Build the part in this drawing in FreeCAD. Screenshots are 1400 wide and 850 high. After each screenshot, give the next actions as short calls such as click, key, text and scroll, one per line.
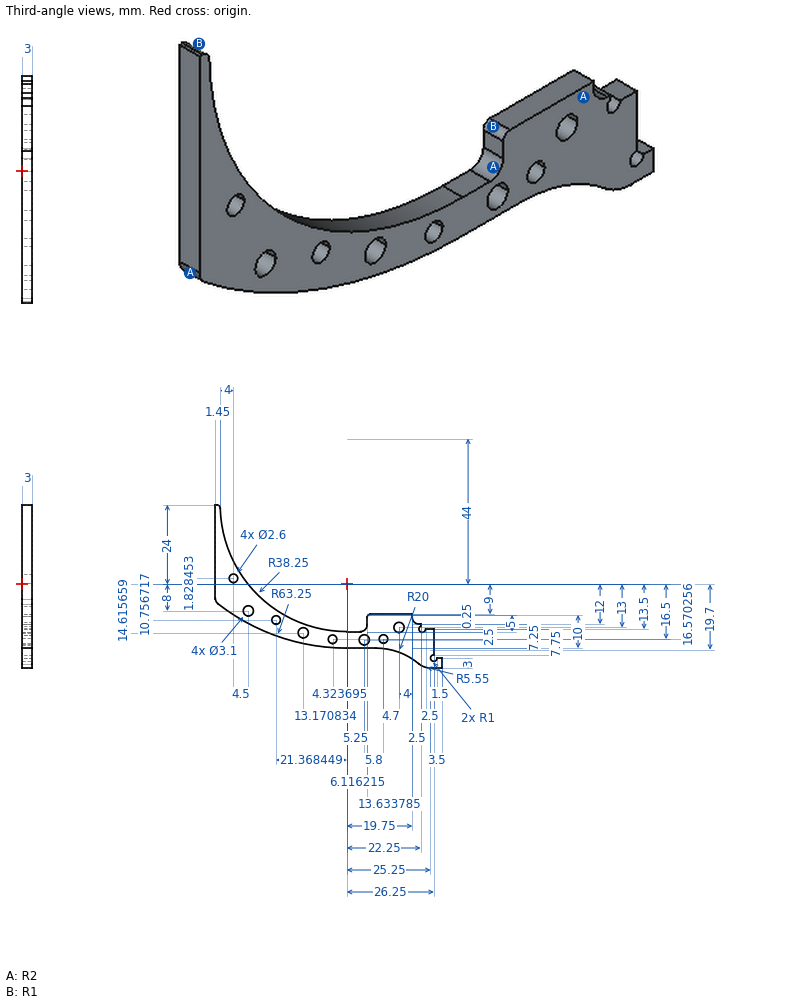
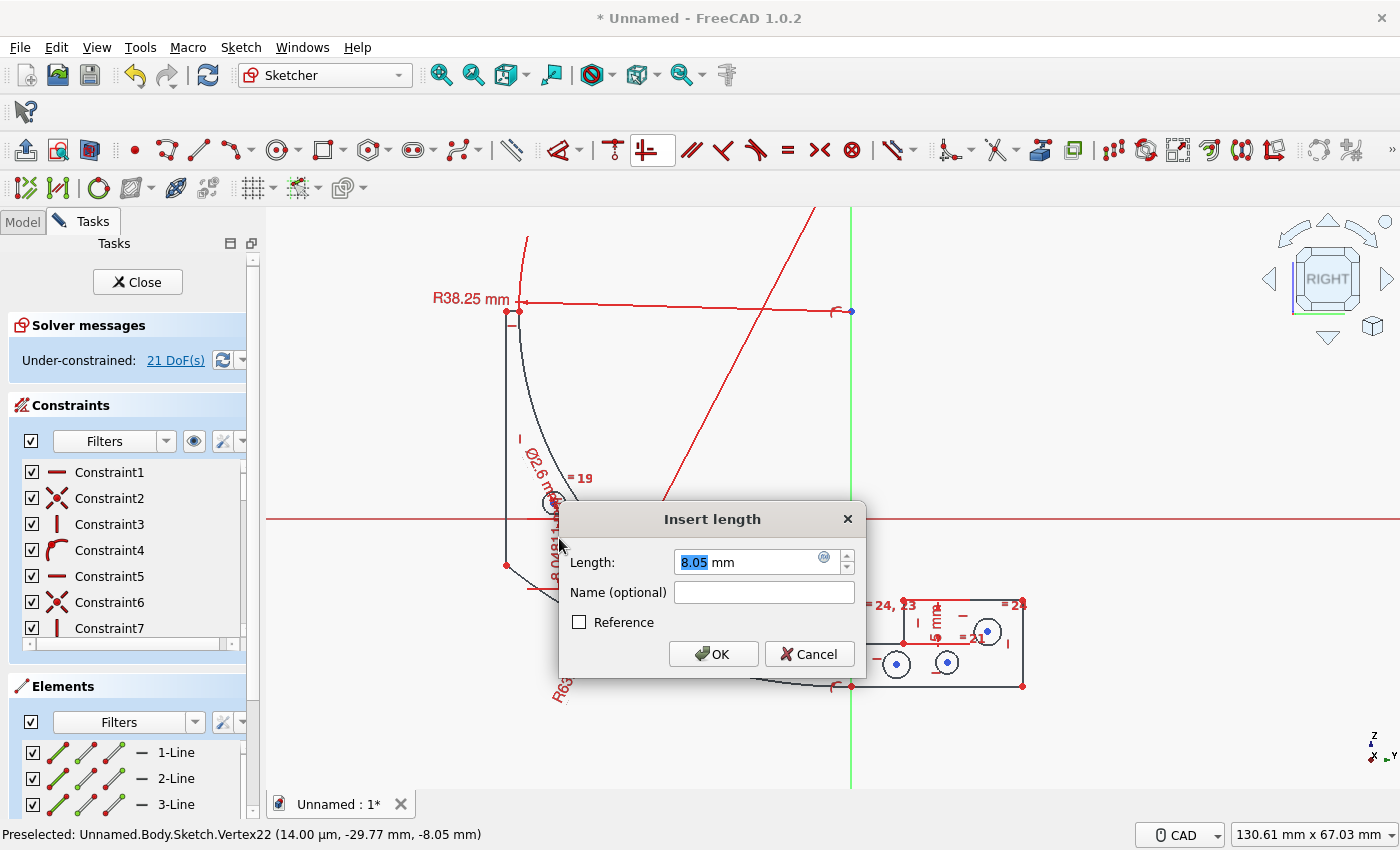
text(8)
key(Return)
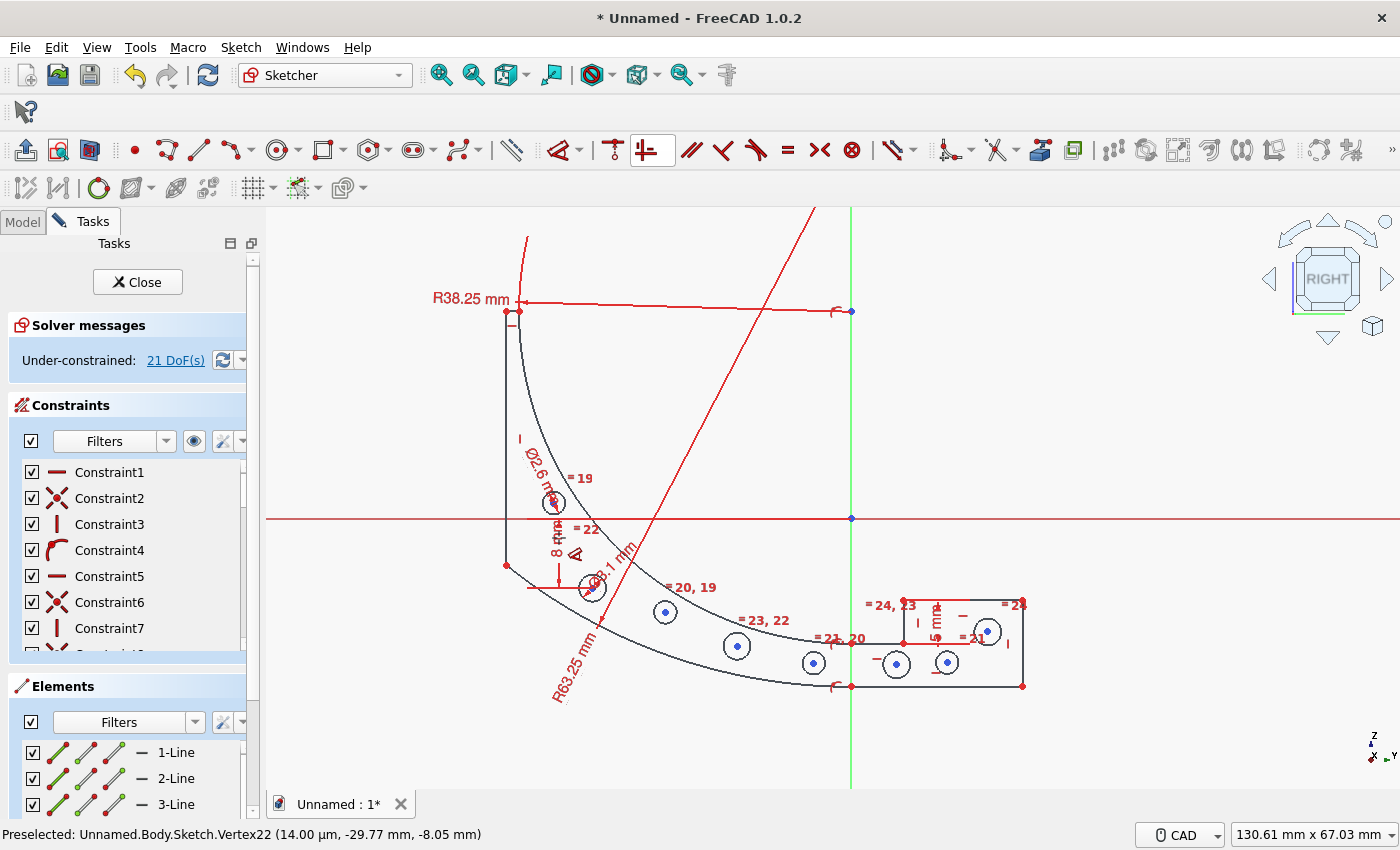
click(1023, 661)
click(1057, 644)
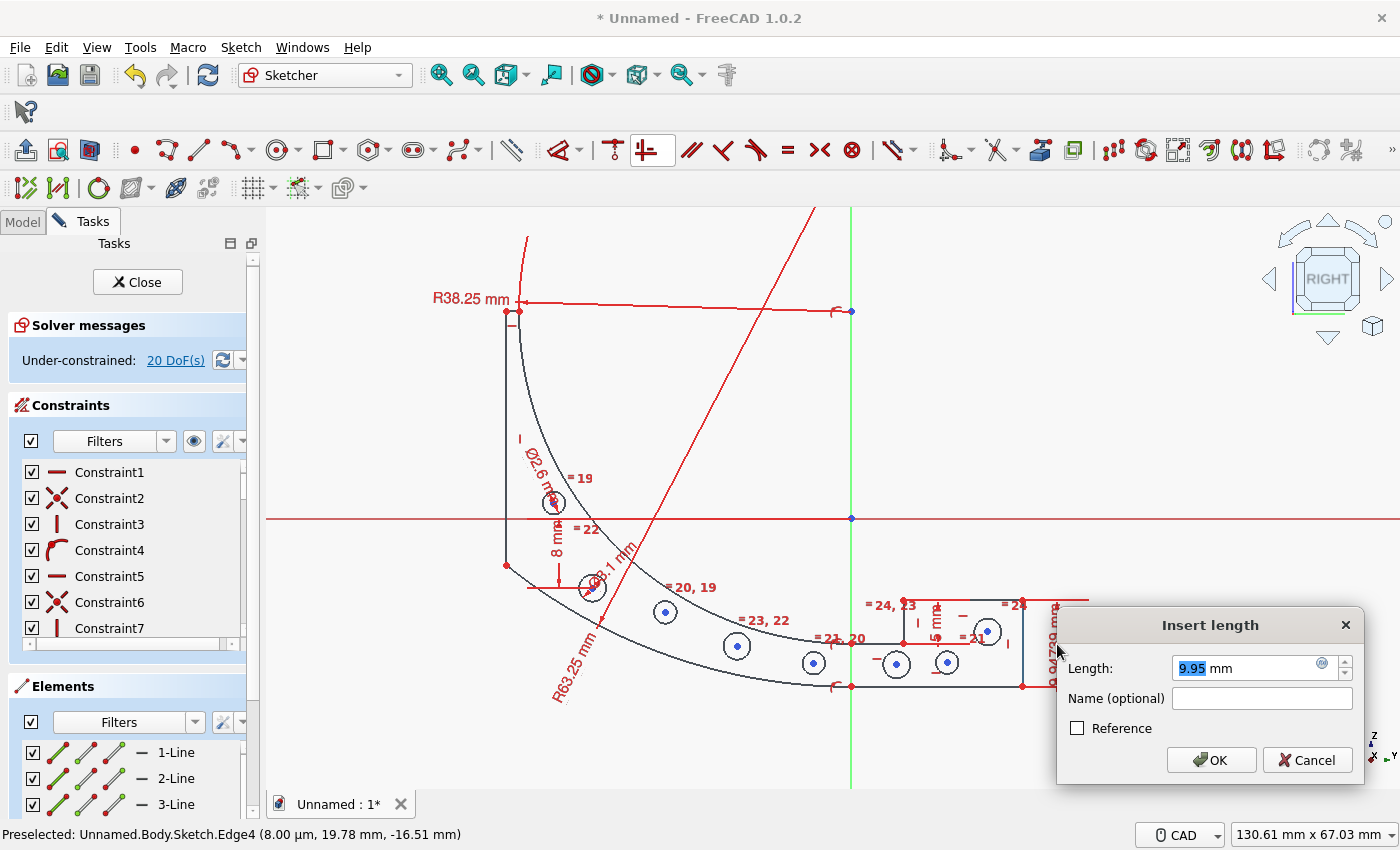
text(10)
key(Return)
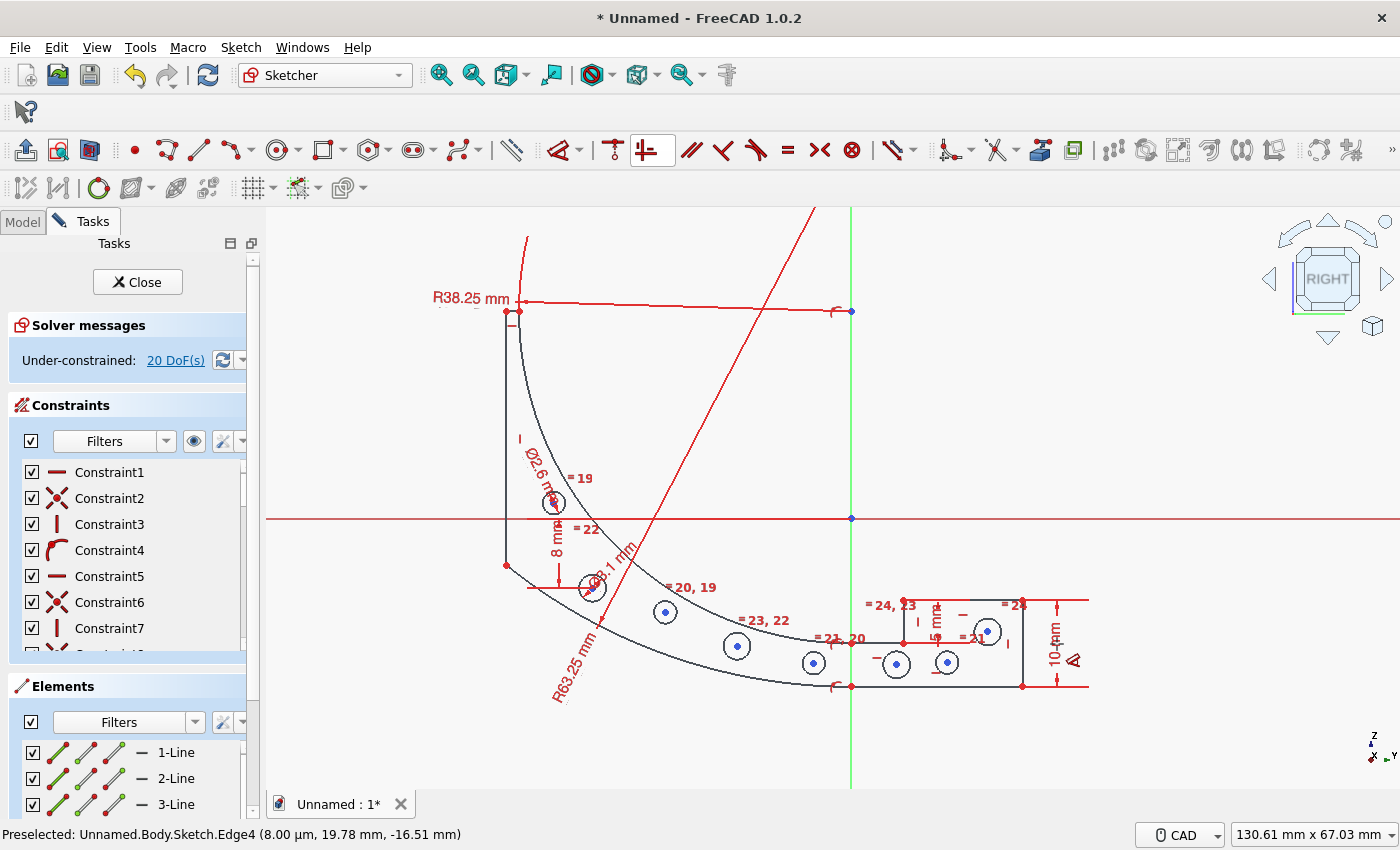
click(988, 632)
click(1022, 575)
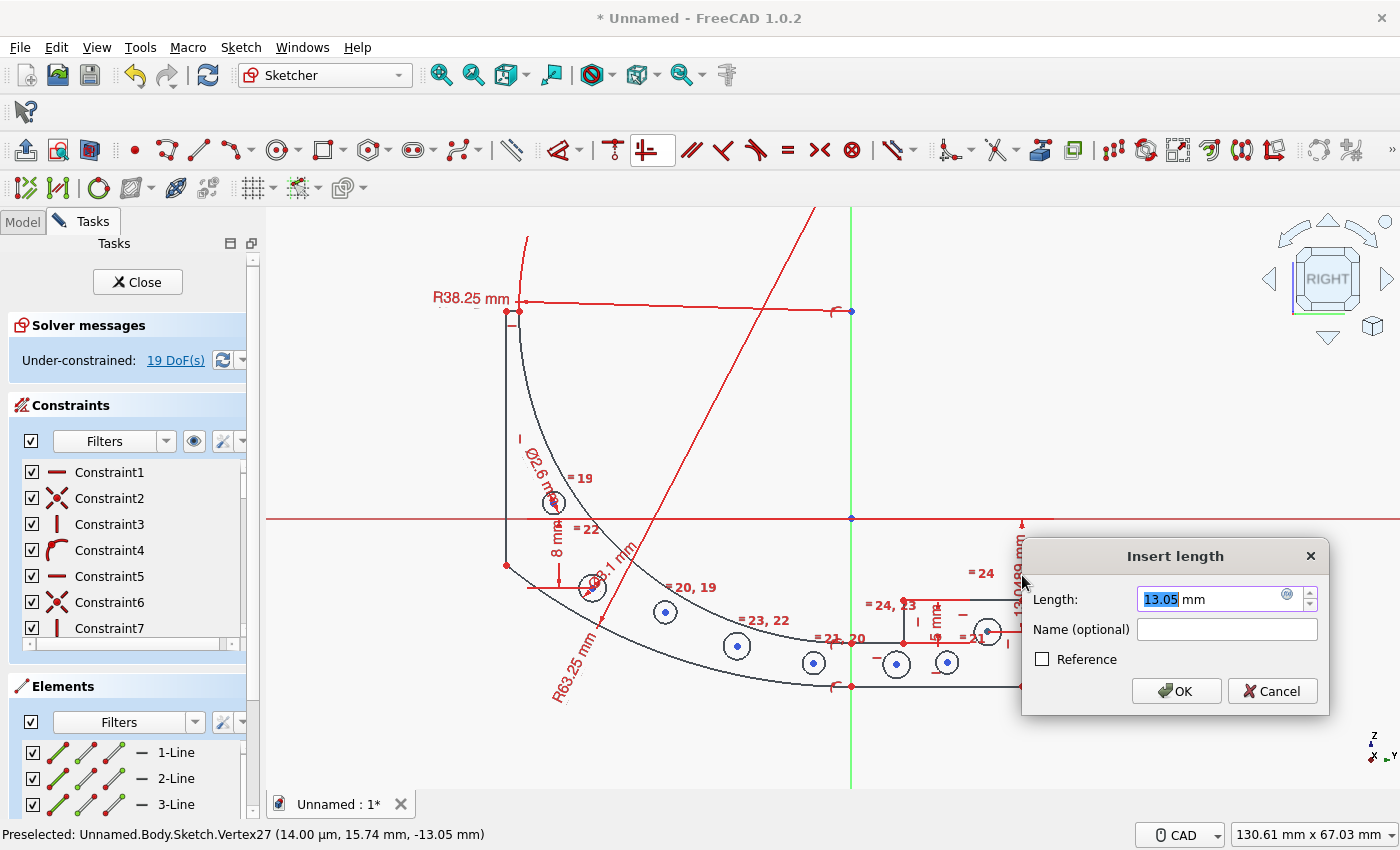
text(13)
key(Return)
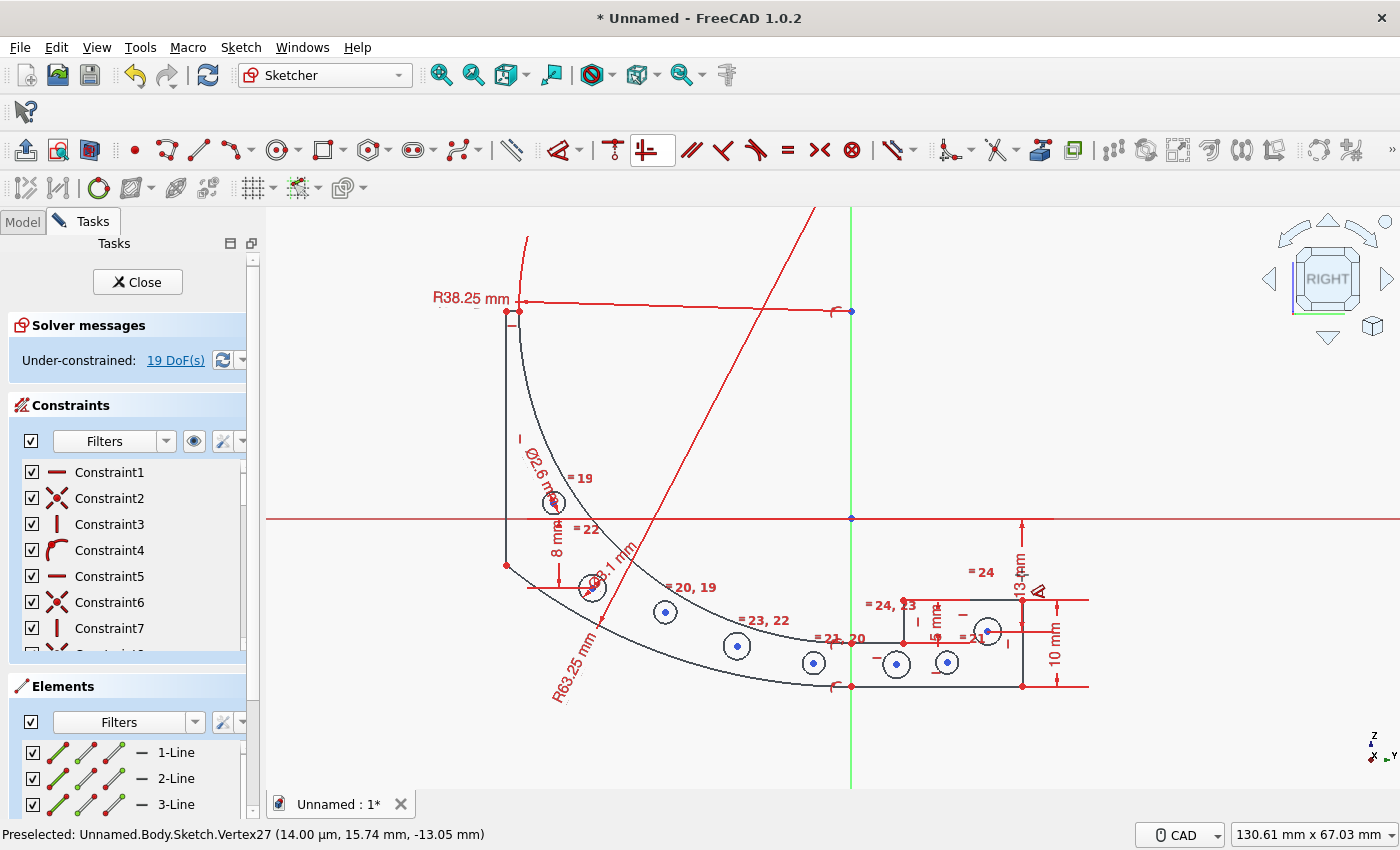
click(519, 311)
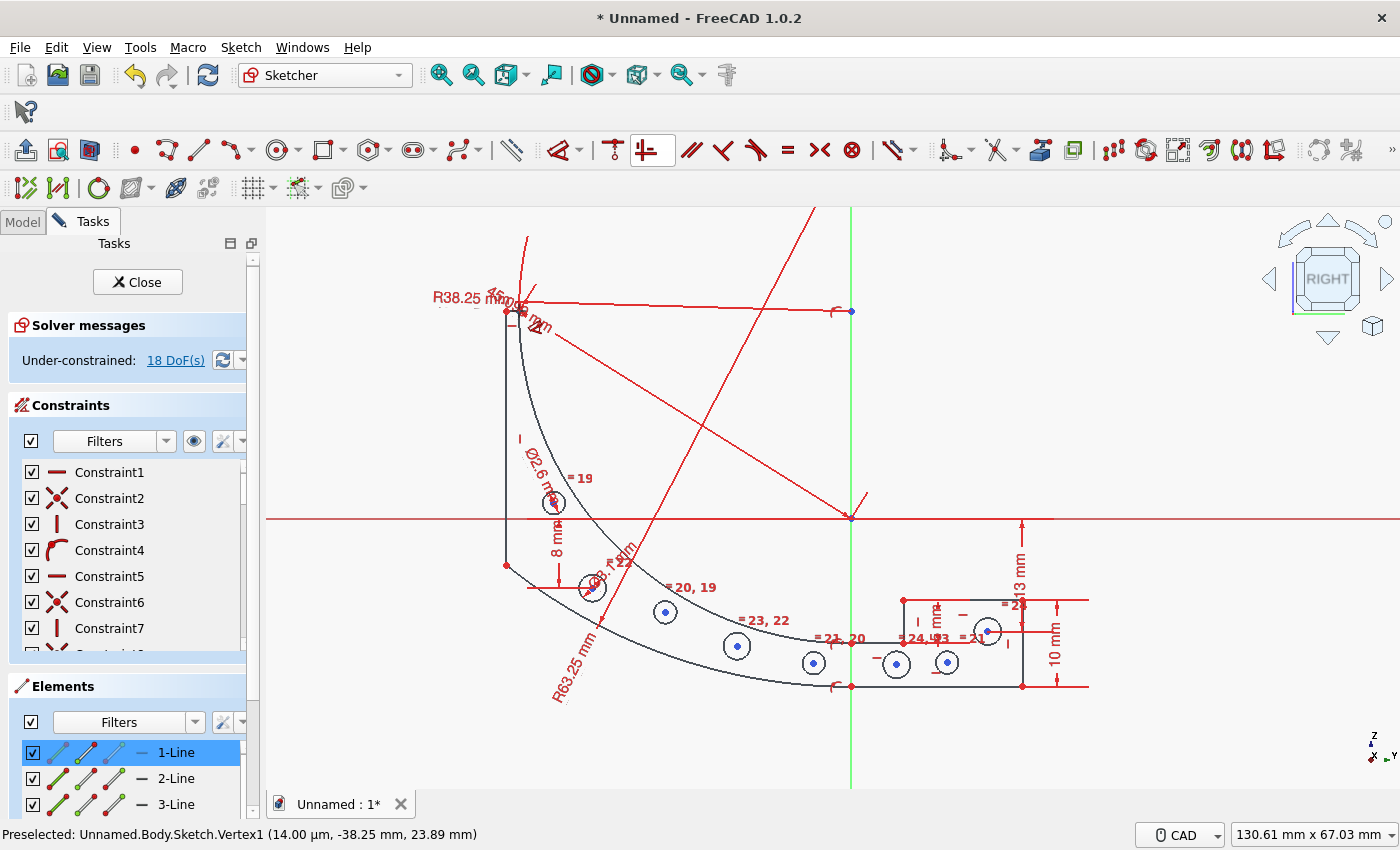
click(554, 503)
click(536, 277)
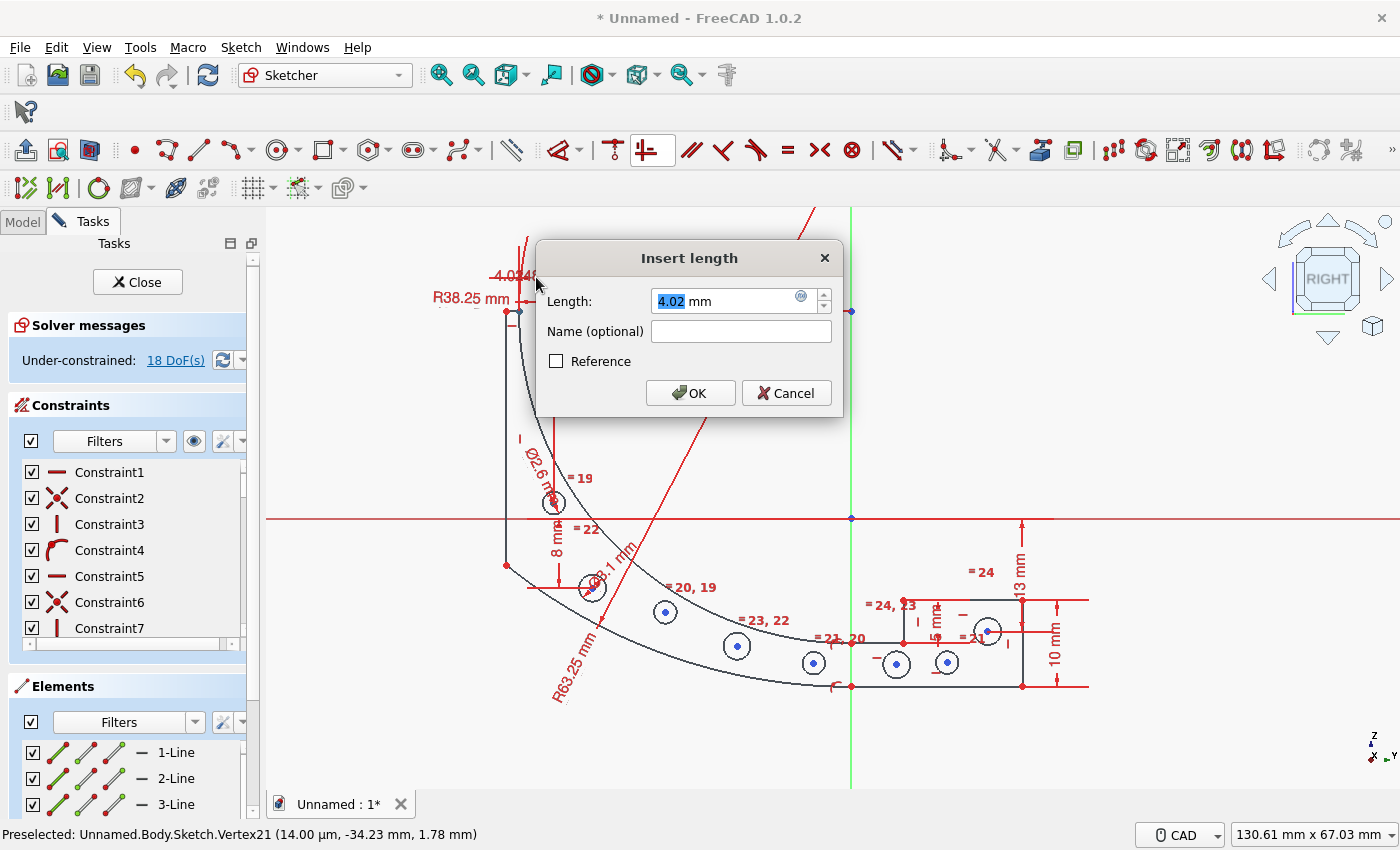
text(4)
key(Return)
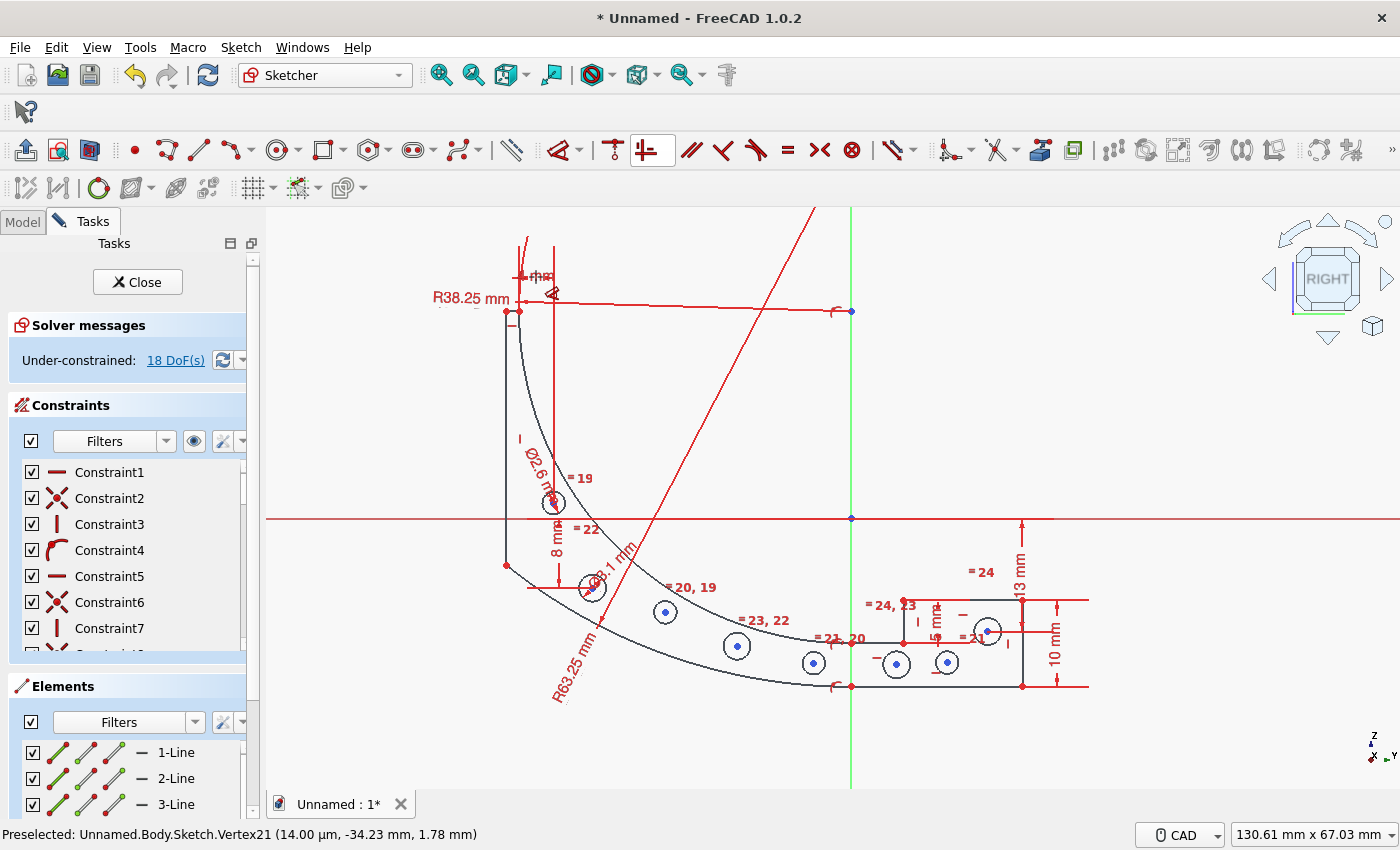
click(1023, 600)